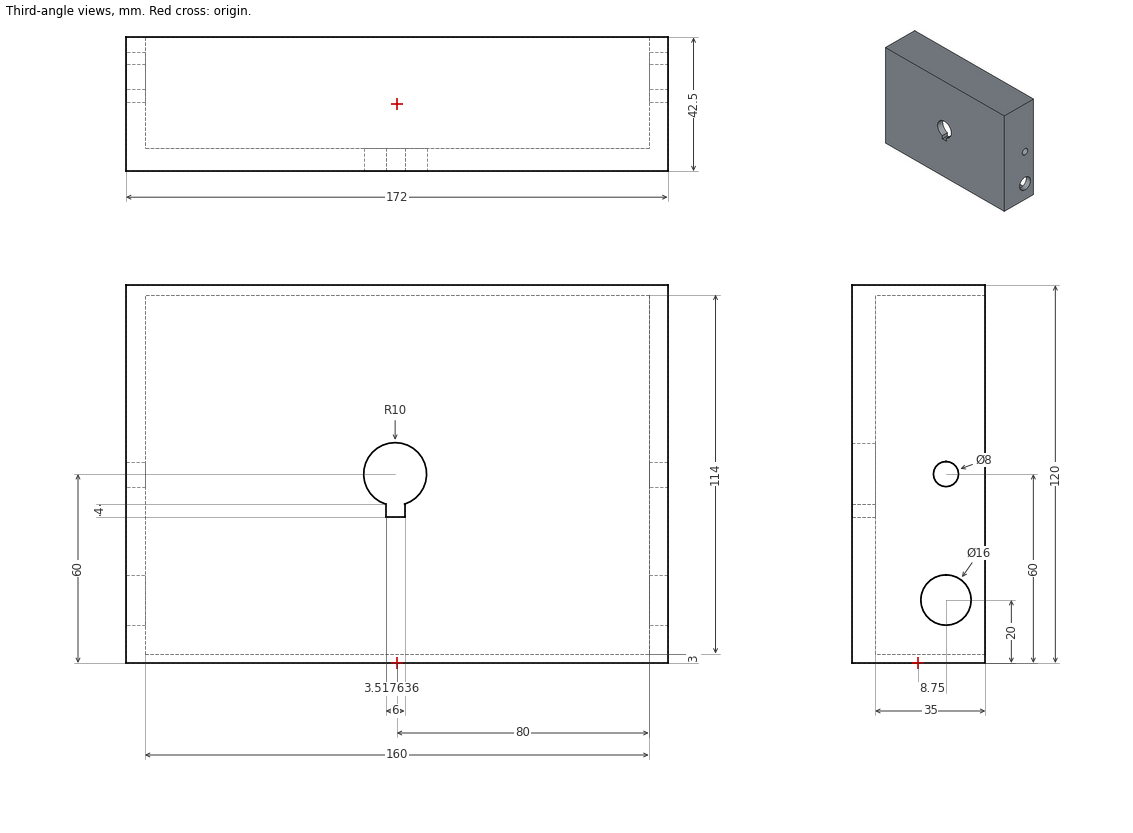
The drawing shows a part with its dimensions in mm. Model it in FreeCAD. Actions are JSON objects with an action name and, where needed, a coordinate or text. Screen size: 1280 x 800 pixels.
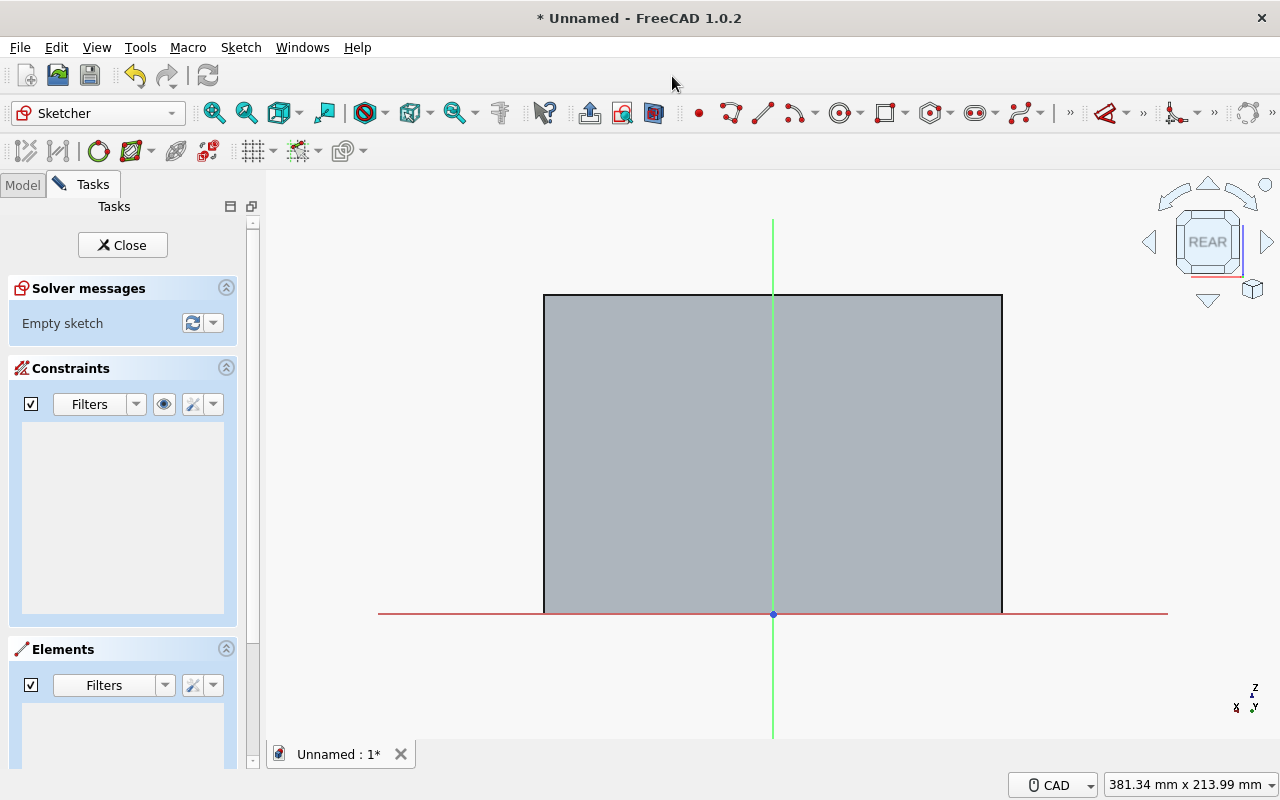
{"action": "left_click", "coordinate": [886, 114]}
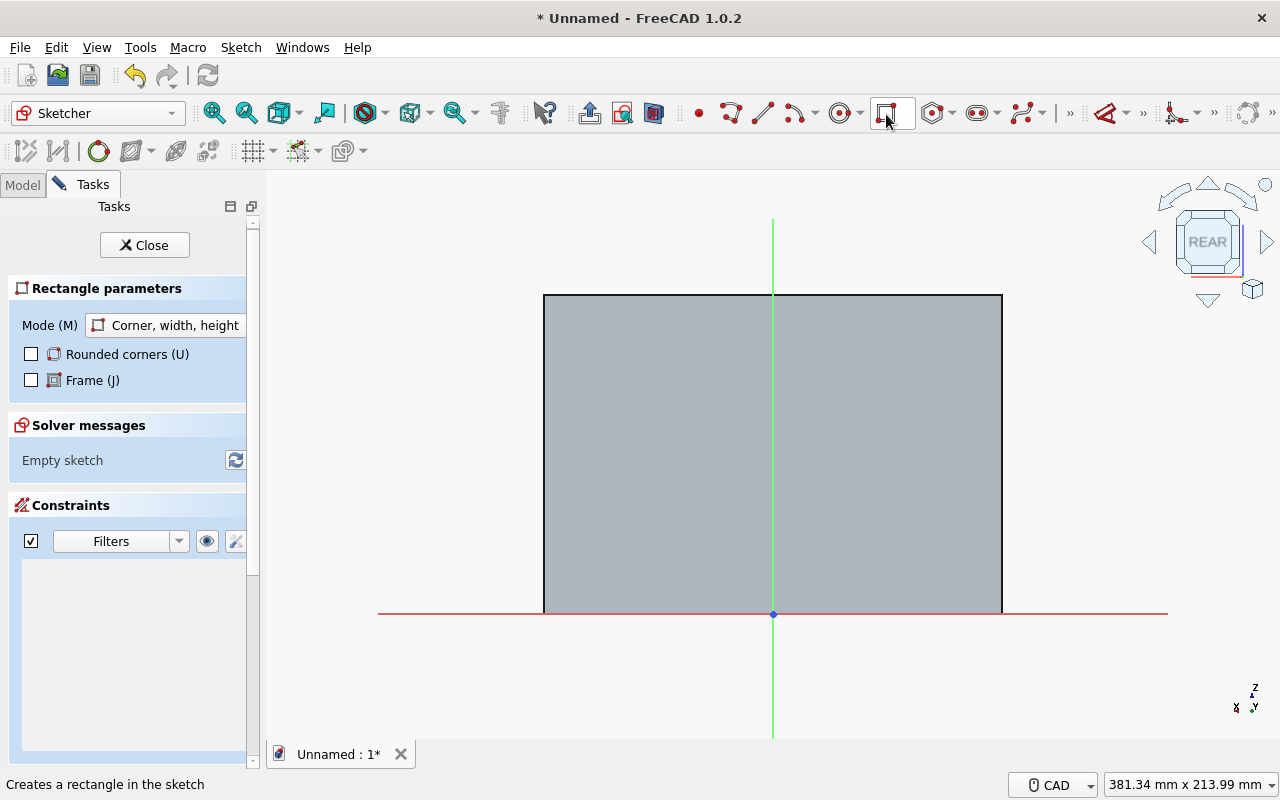
{"action": "left_click", "coordinate": [560, 303]}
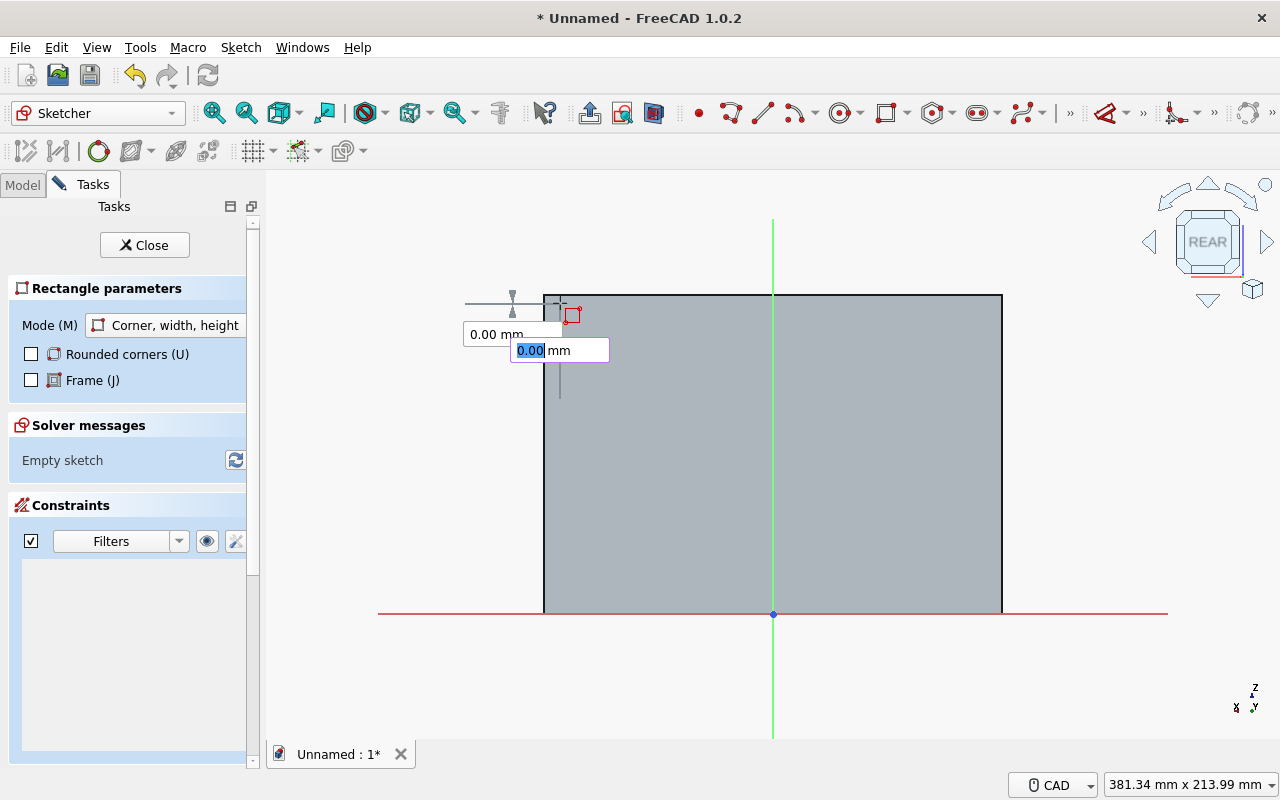
{"action": "scroll", "coordinate": [986, 606], "scroll_direction": "up", "scroll_amount": 4}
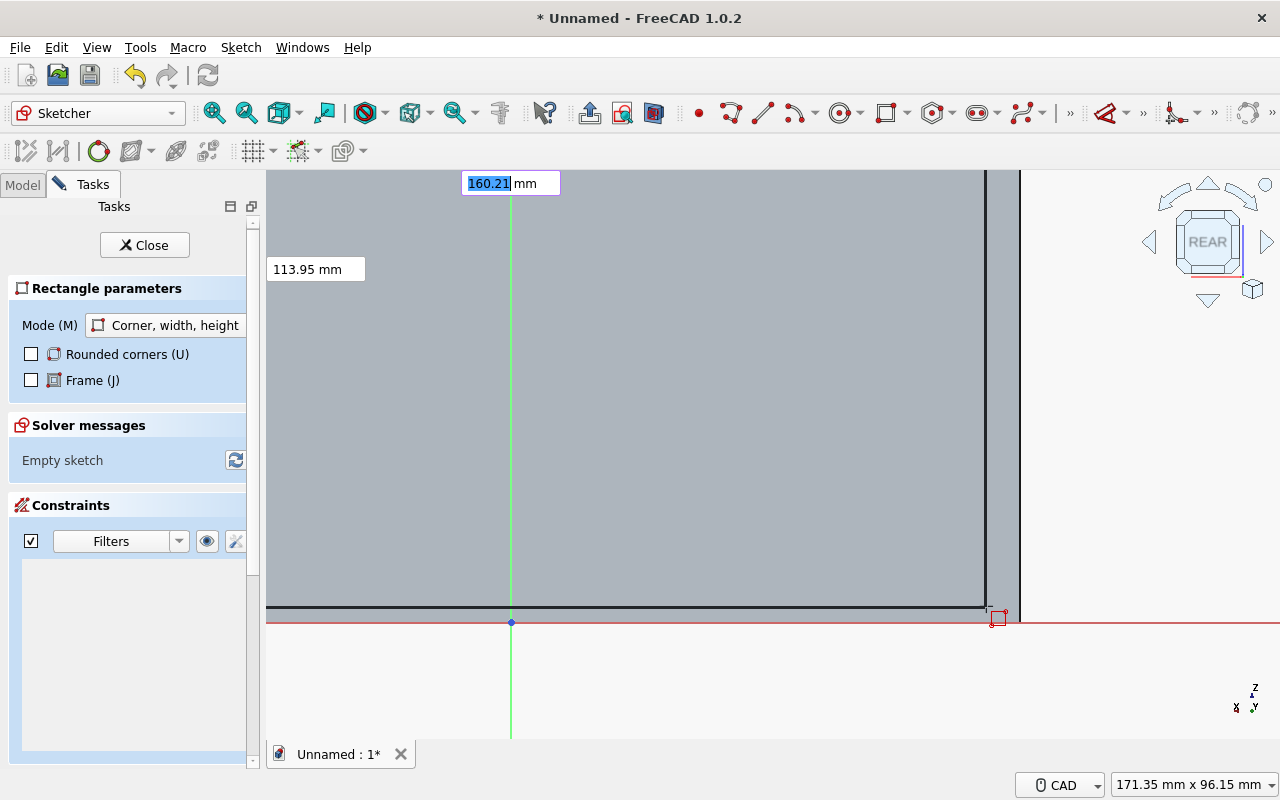
{"action": "left_click", "coordinate": [985, 605]}
{"action": "key", "text": "Escape"}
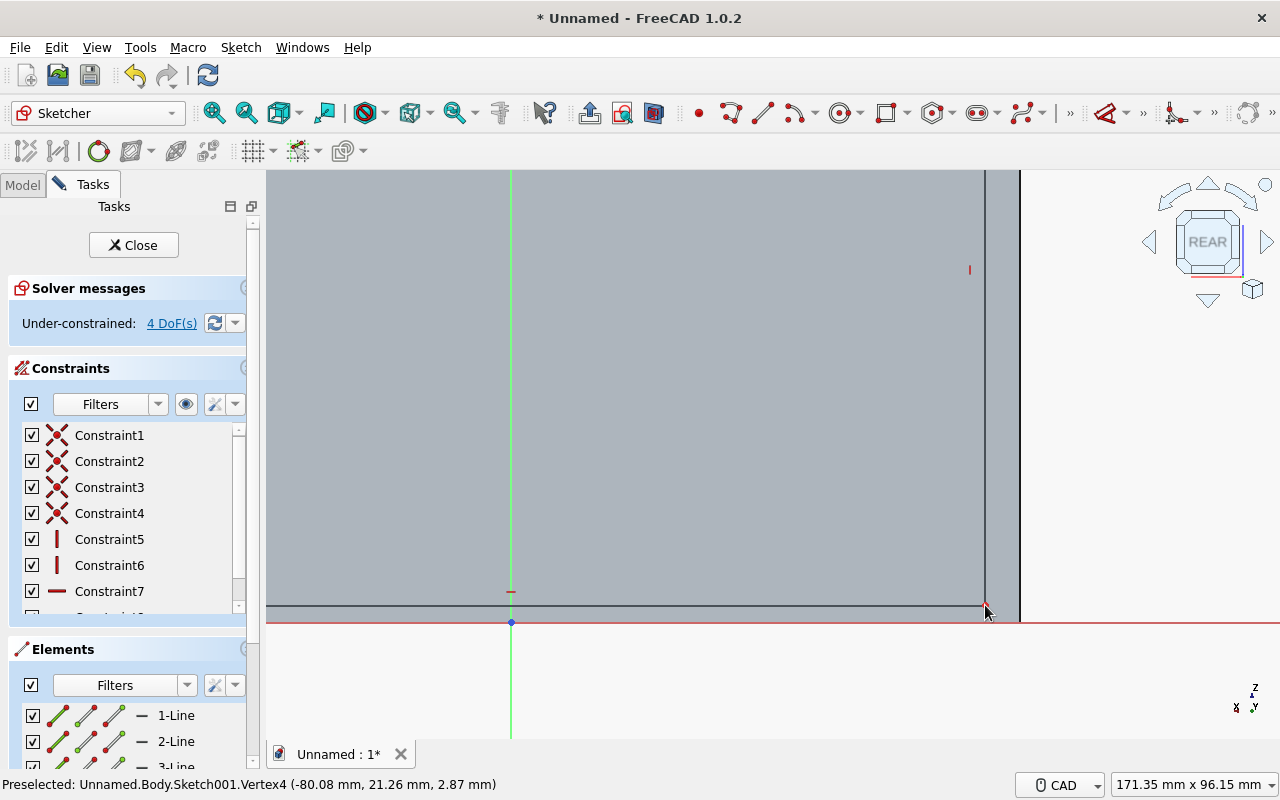
{"action": "left_click", "coordinate": [1106, 114]}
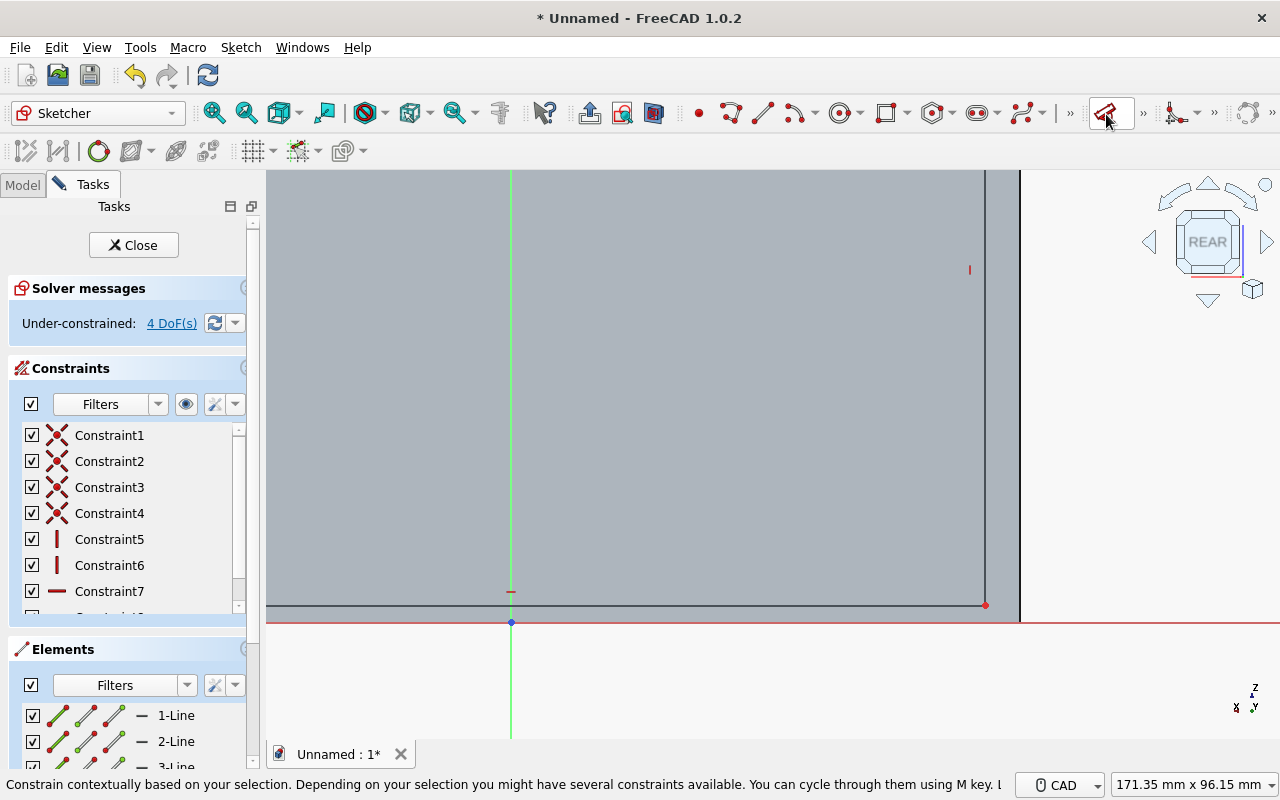
{"action": "scroll", "coordinate": [940, 671], "scroll_direction": "down", "scroll_amount": 3}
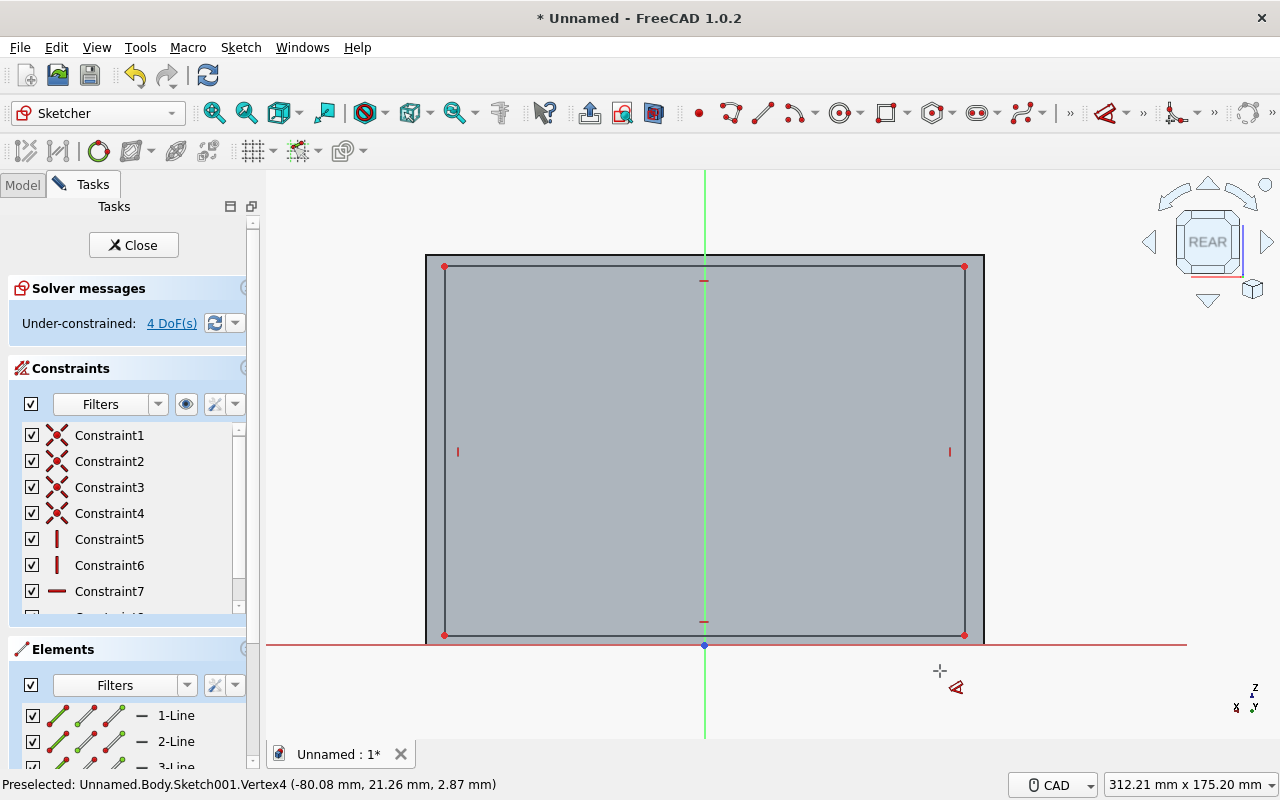
{"action": "scroll", "coordinate": [445, 636], "scroll_direction": "up", "scroll_amount": 8}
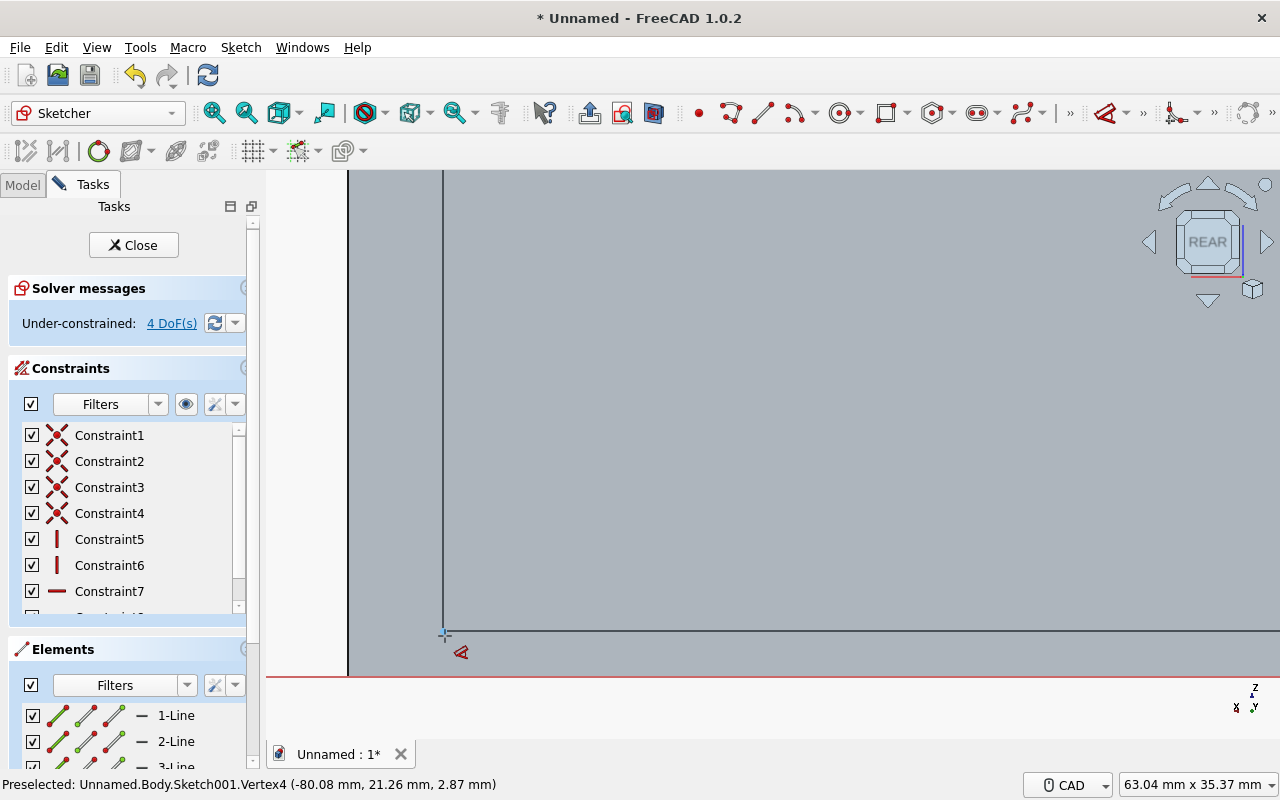
{"action": "left_click", "coordinate": [443, 631]}
{"action": "left_click", "coordinate": [409, 654]}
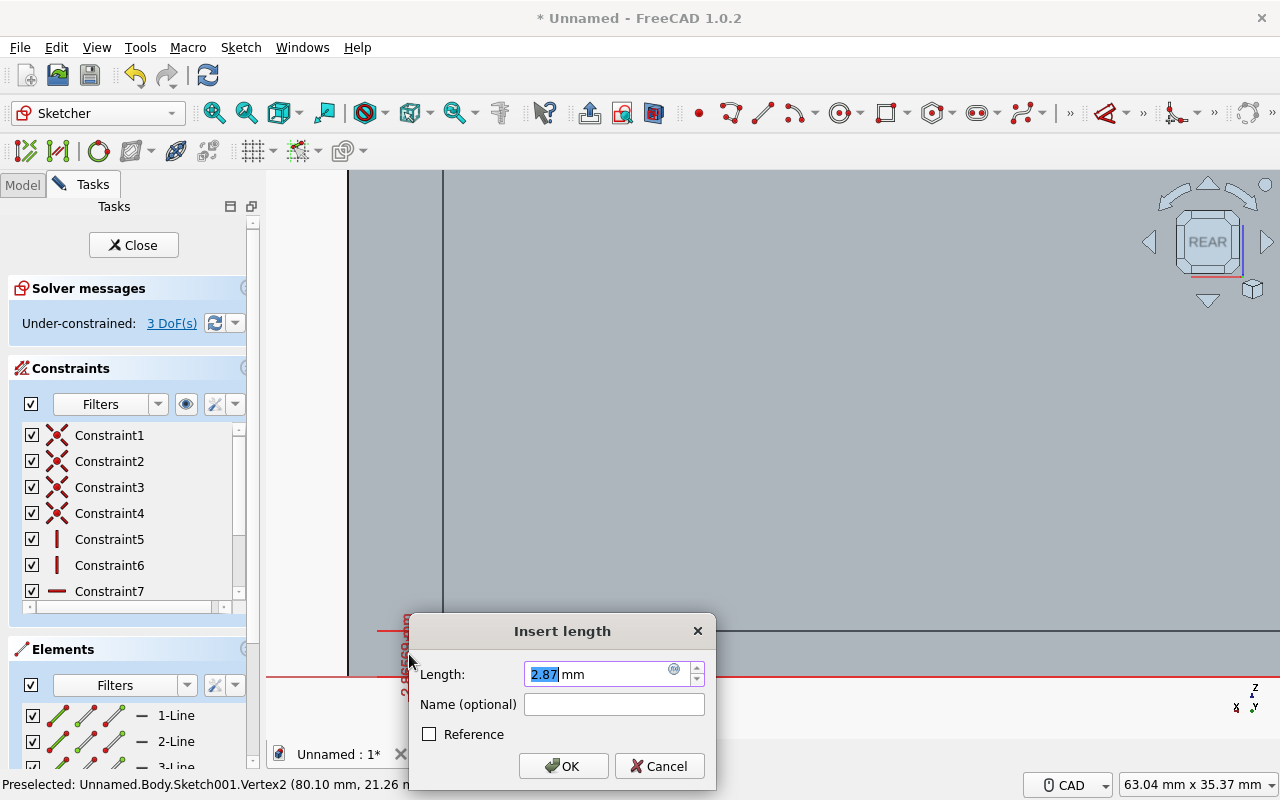
{"action": "type", "text": "3"}
{"action": "key", "text": "Return"}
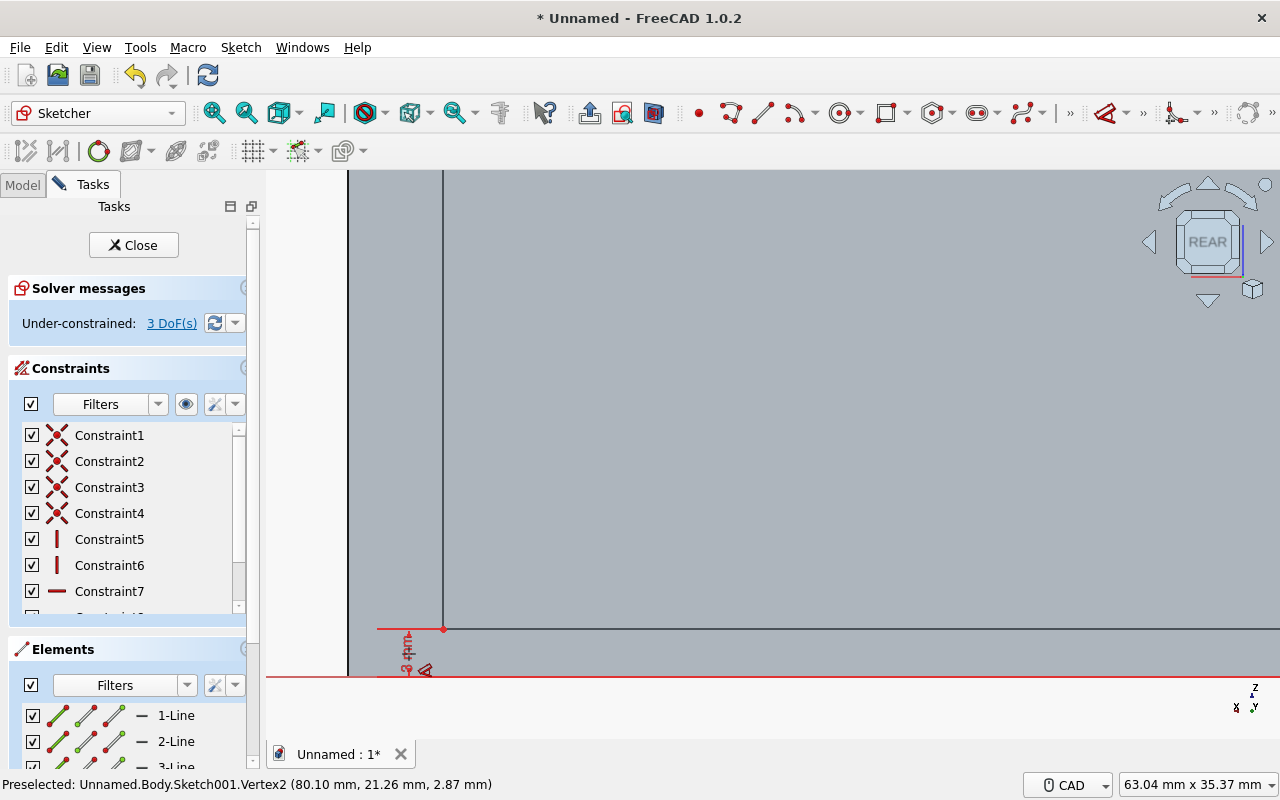
{"action": "scroll", "coordinate": [445, 636], "scroll_direction": "down", "scroll_amount": 8}